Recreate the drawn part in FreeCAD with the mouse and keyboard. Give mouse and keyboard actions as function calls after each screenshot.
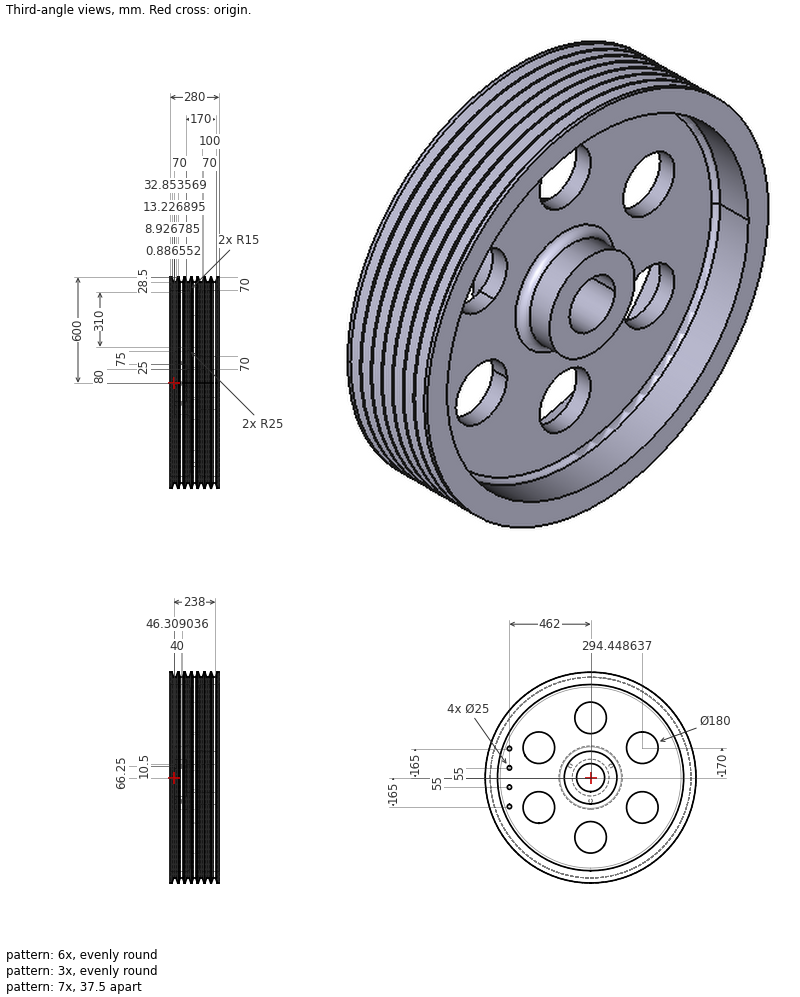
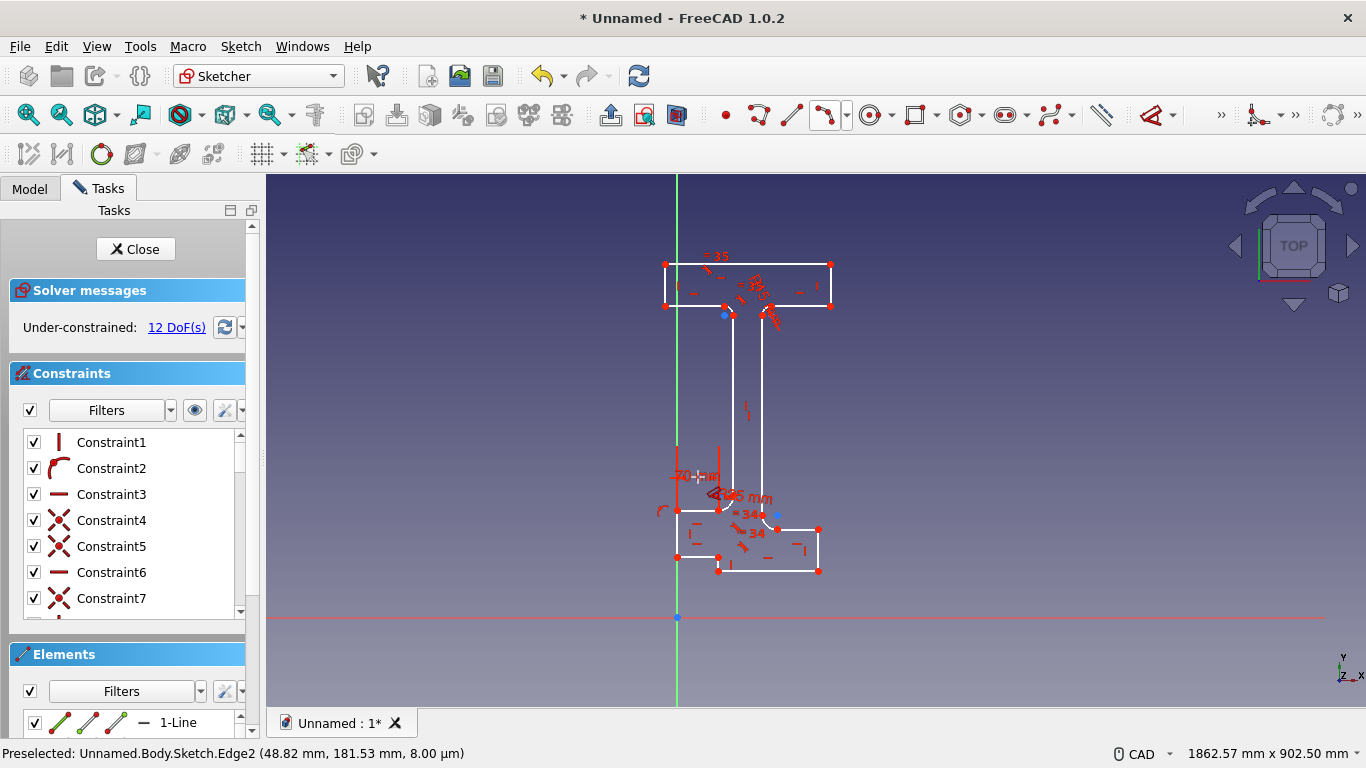
click(677, 525)
click(643, 534)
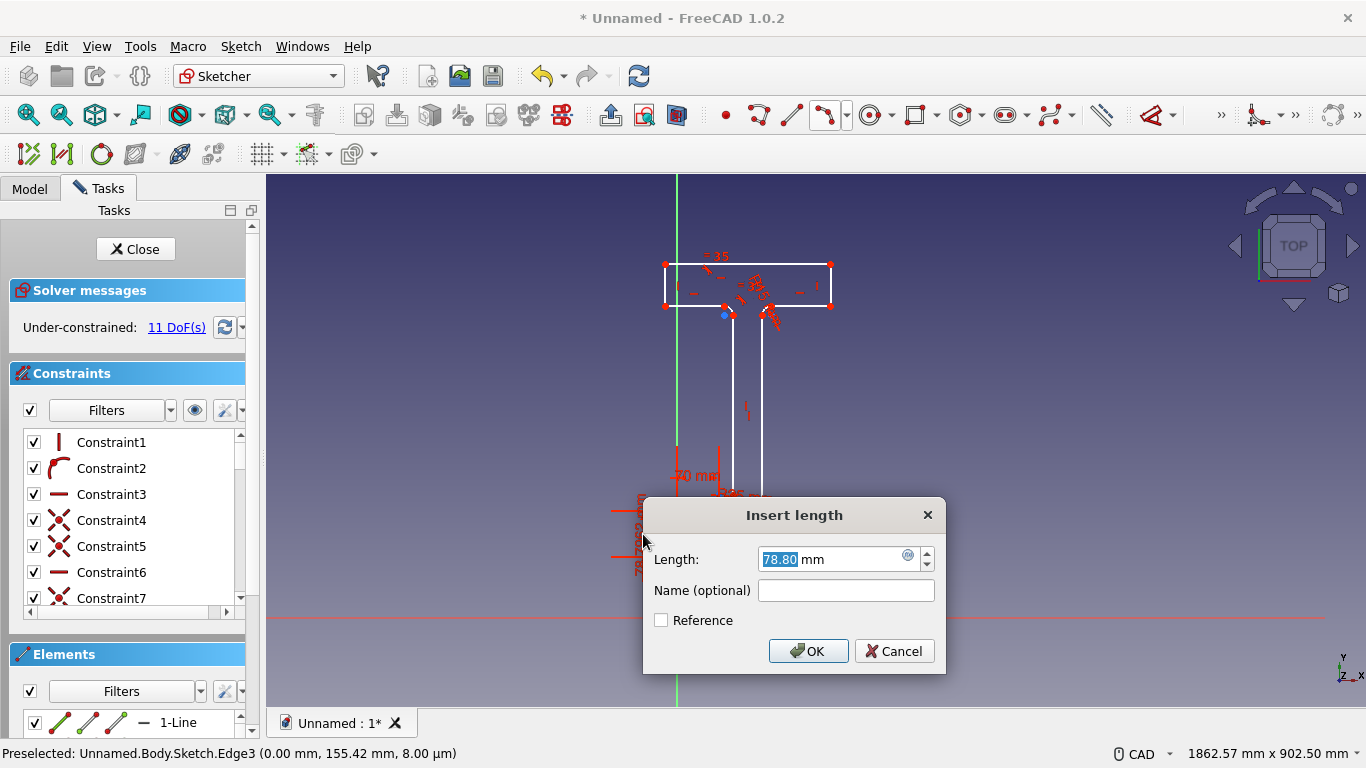
text(75)
key(Return)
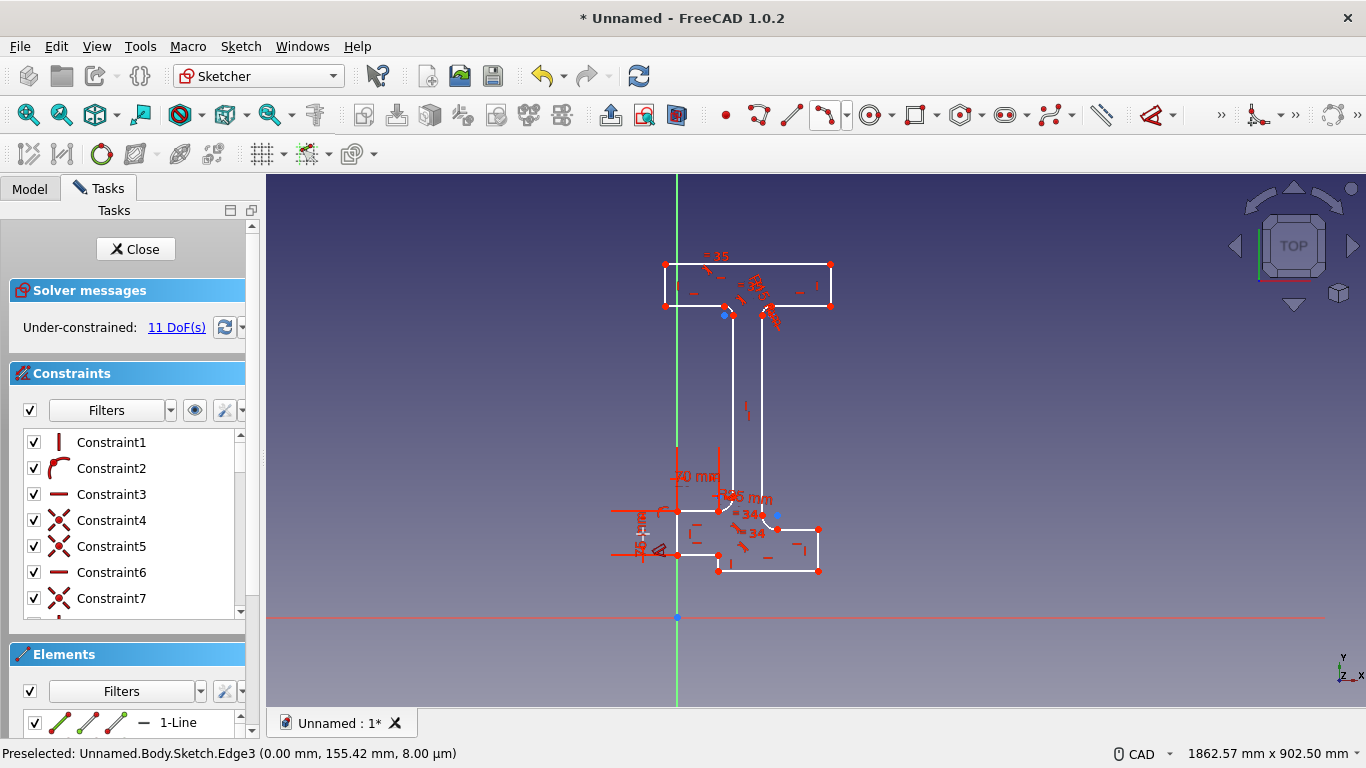
click(690, 555)
click(698, 589)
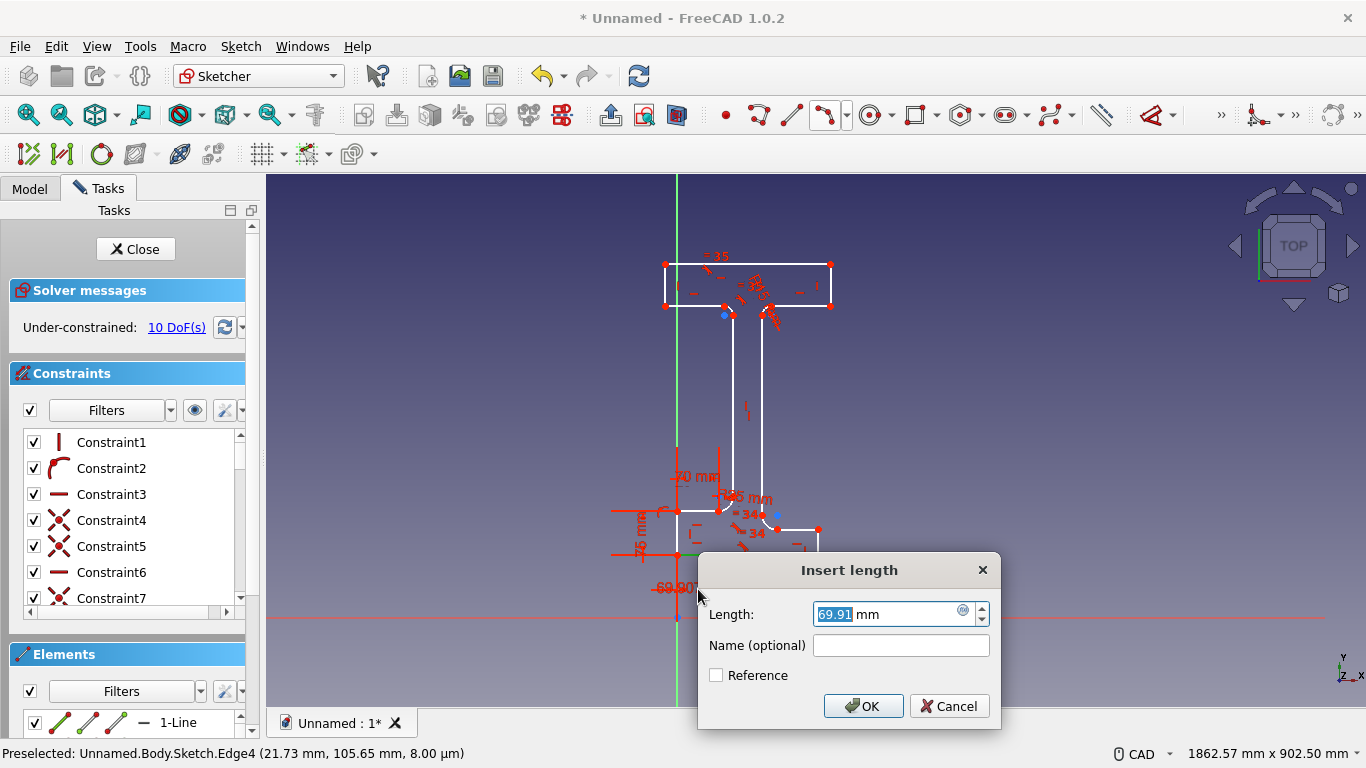
text(70)
key(Return)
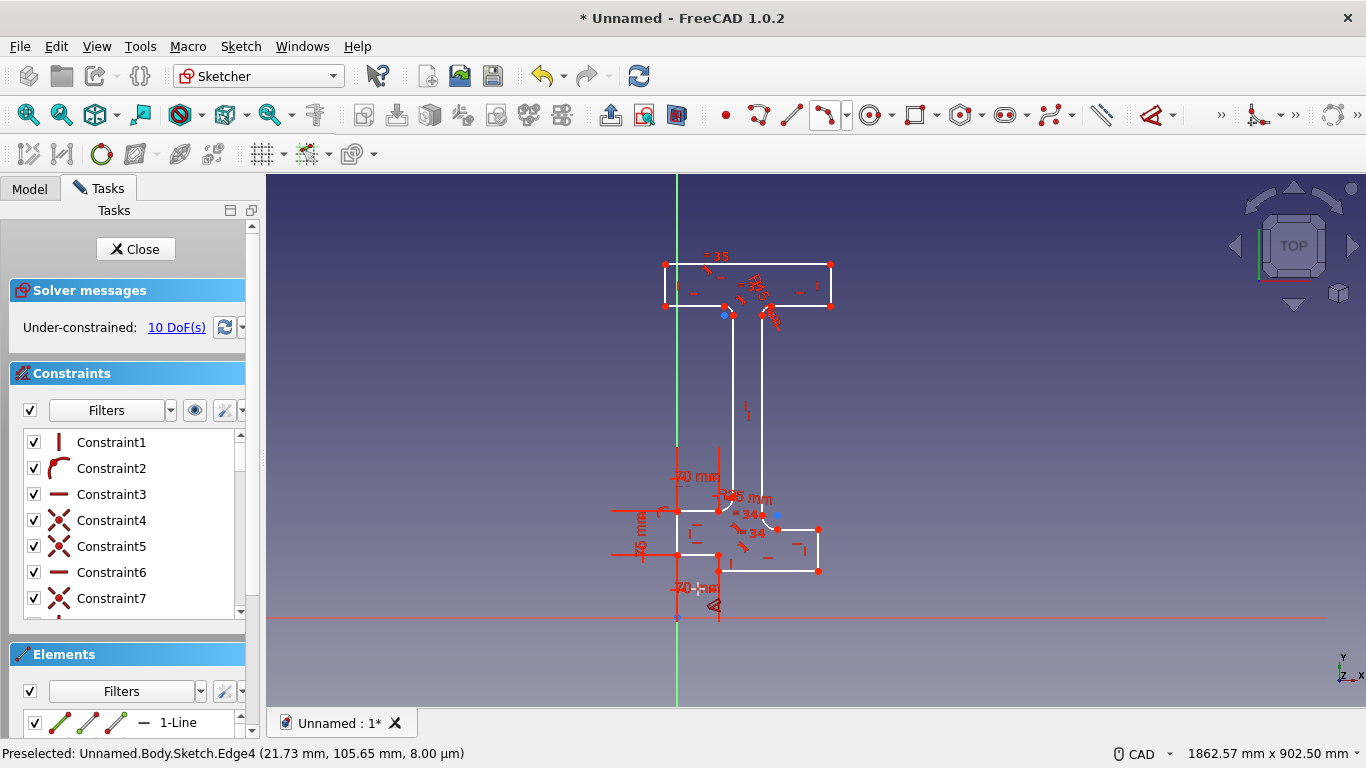
scroll(719, 563, up, 5)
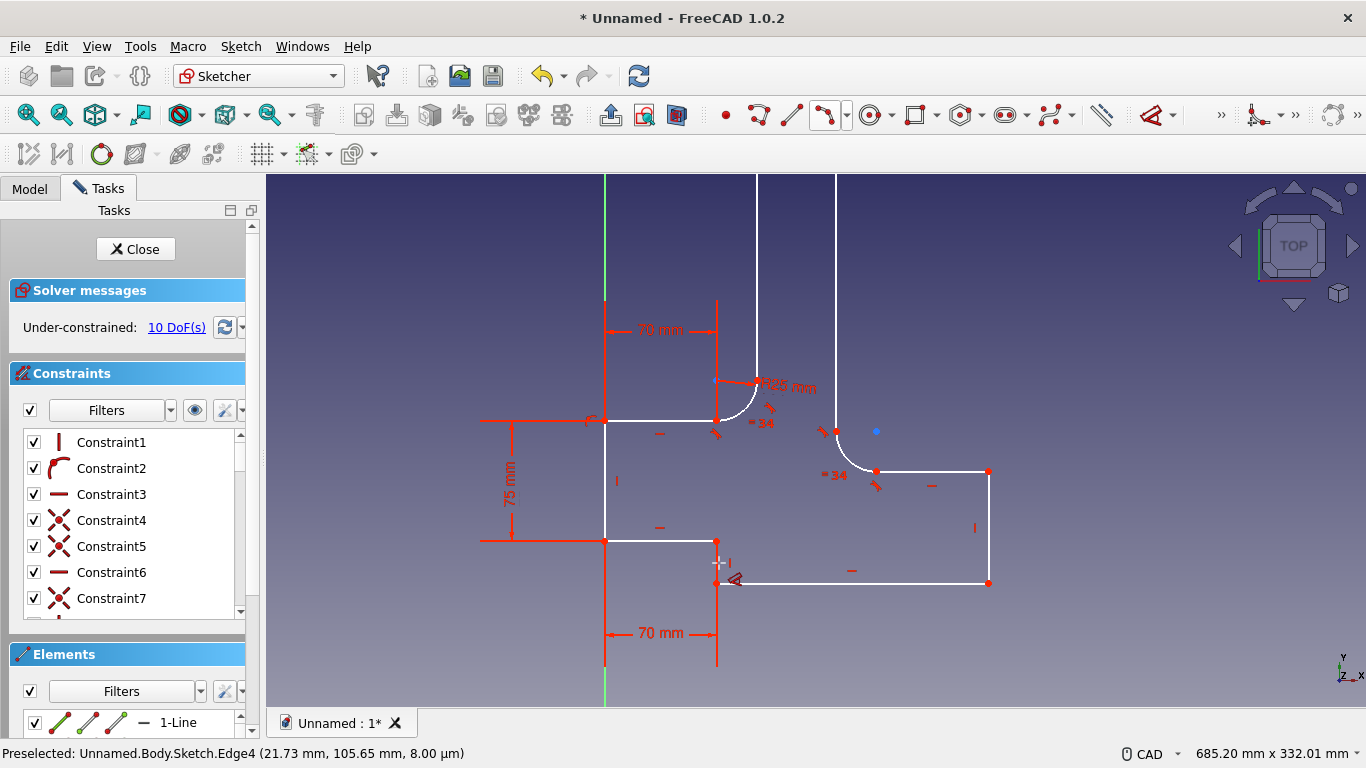
click(717, 562)
click(683, 562)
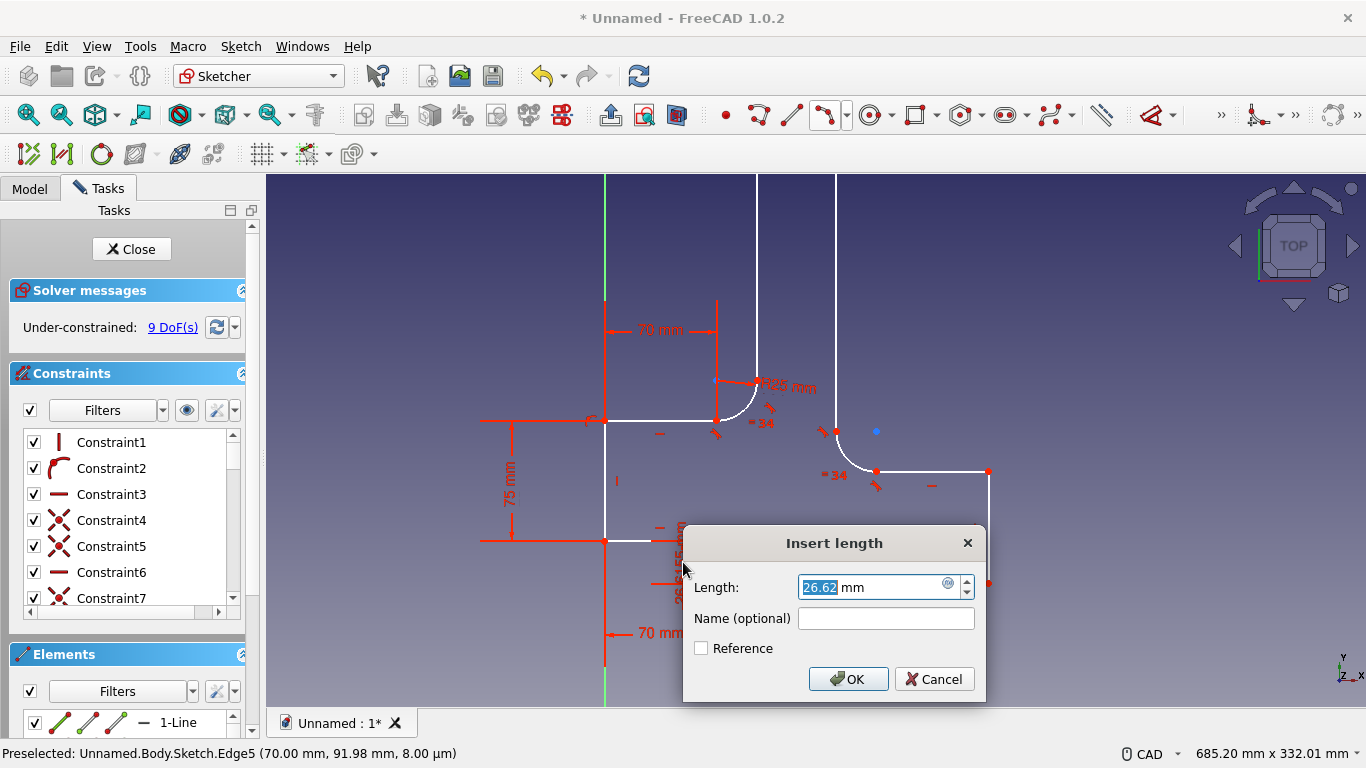
text(25)
key(Return)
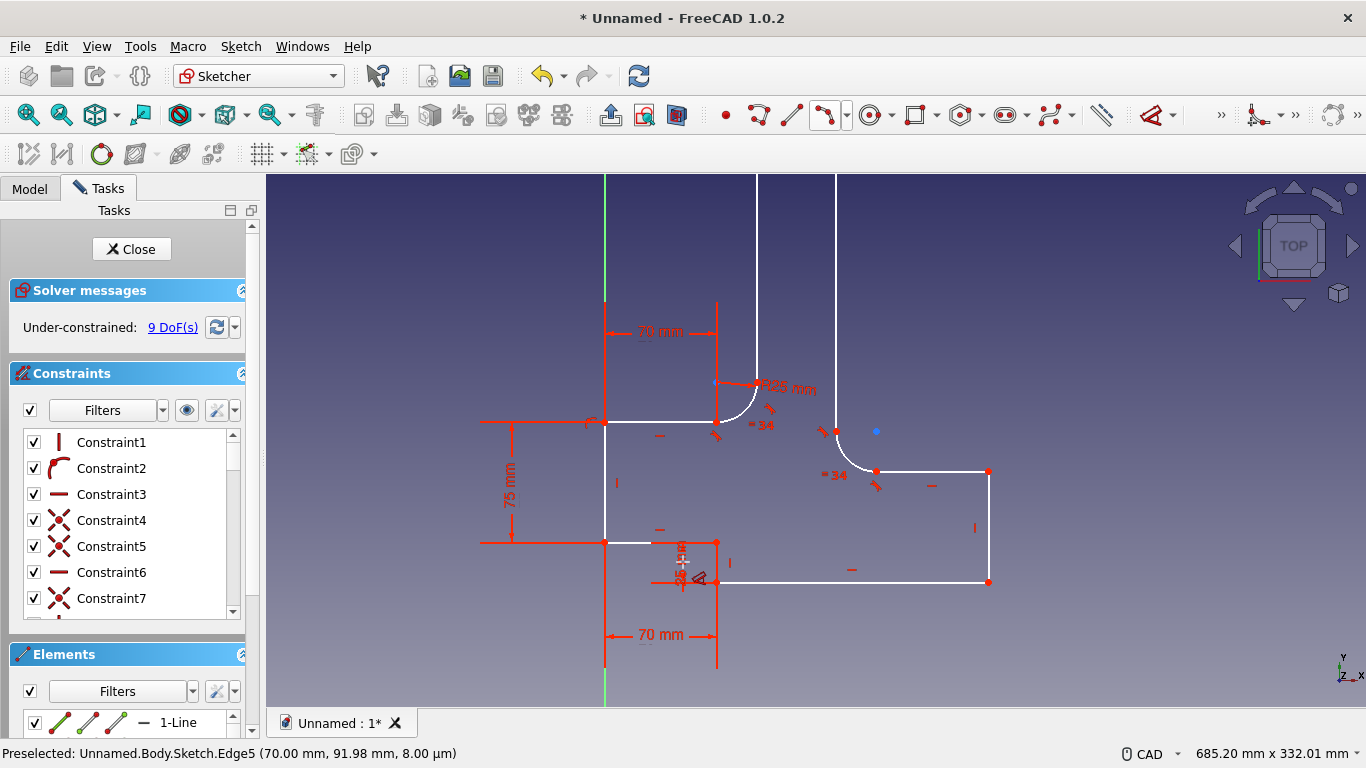
click(989, 549)
click(1023, 527)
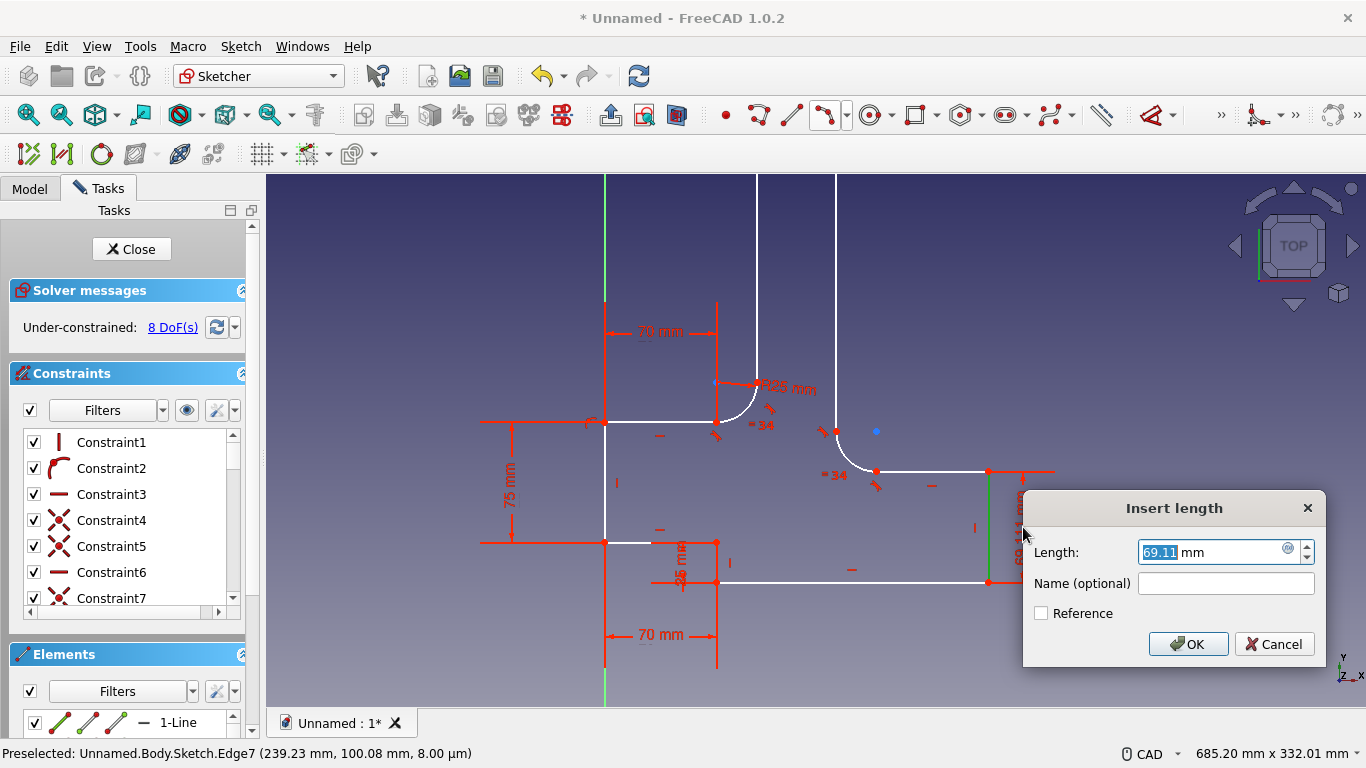
text(70)
key(Return)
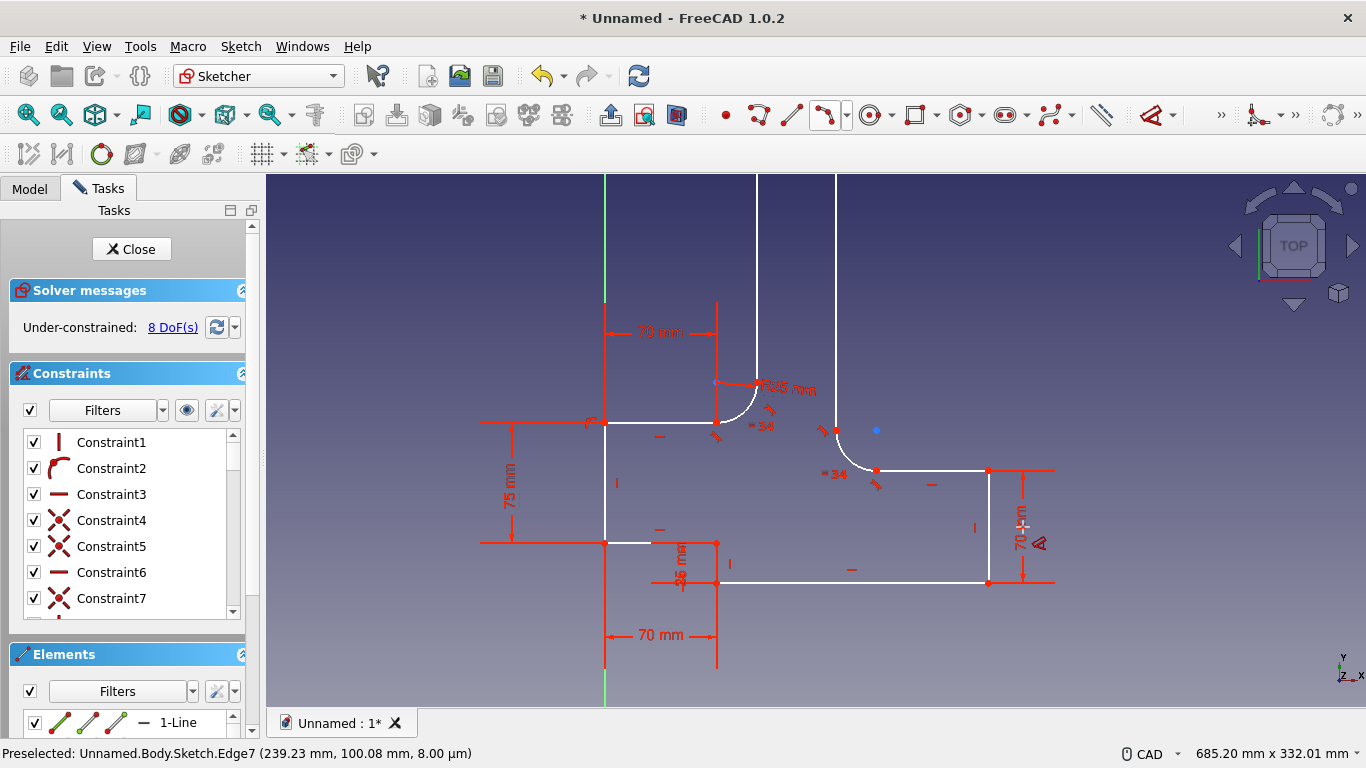
click(955, 471)
click(933, 505)